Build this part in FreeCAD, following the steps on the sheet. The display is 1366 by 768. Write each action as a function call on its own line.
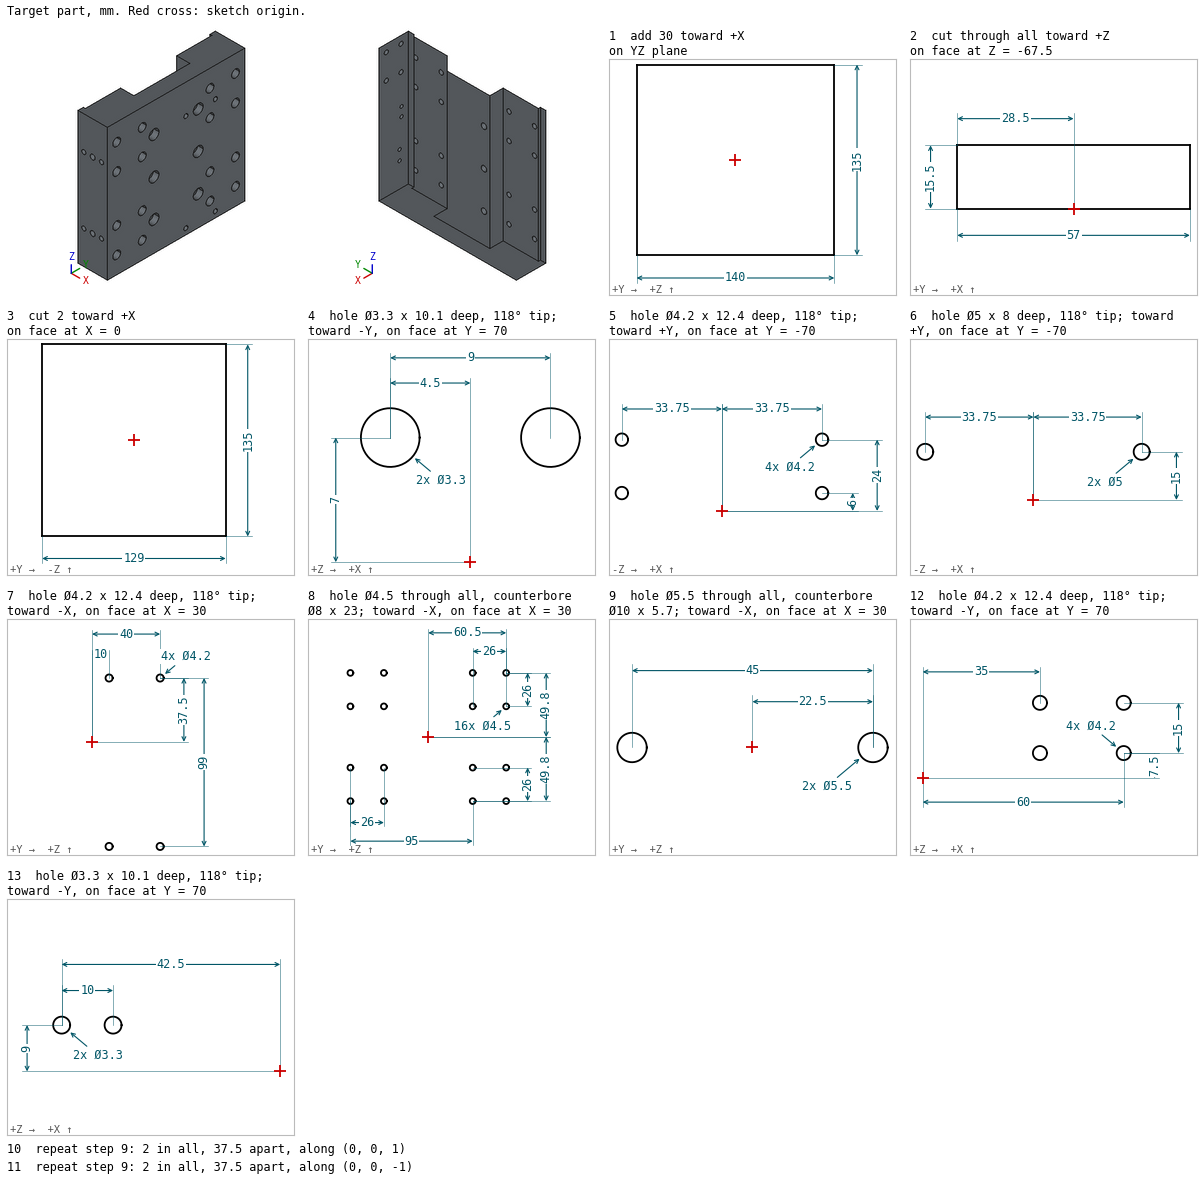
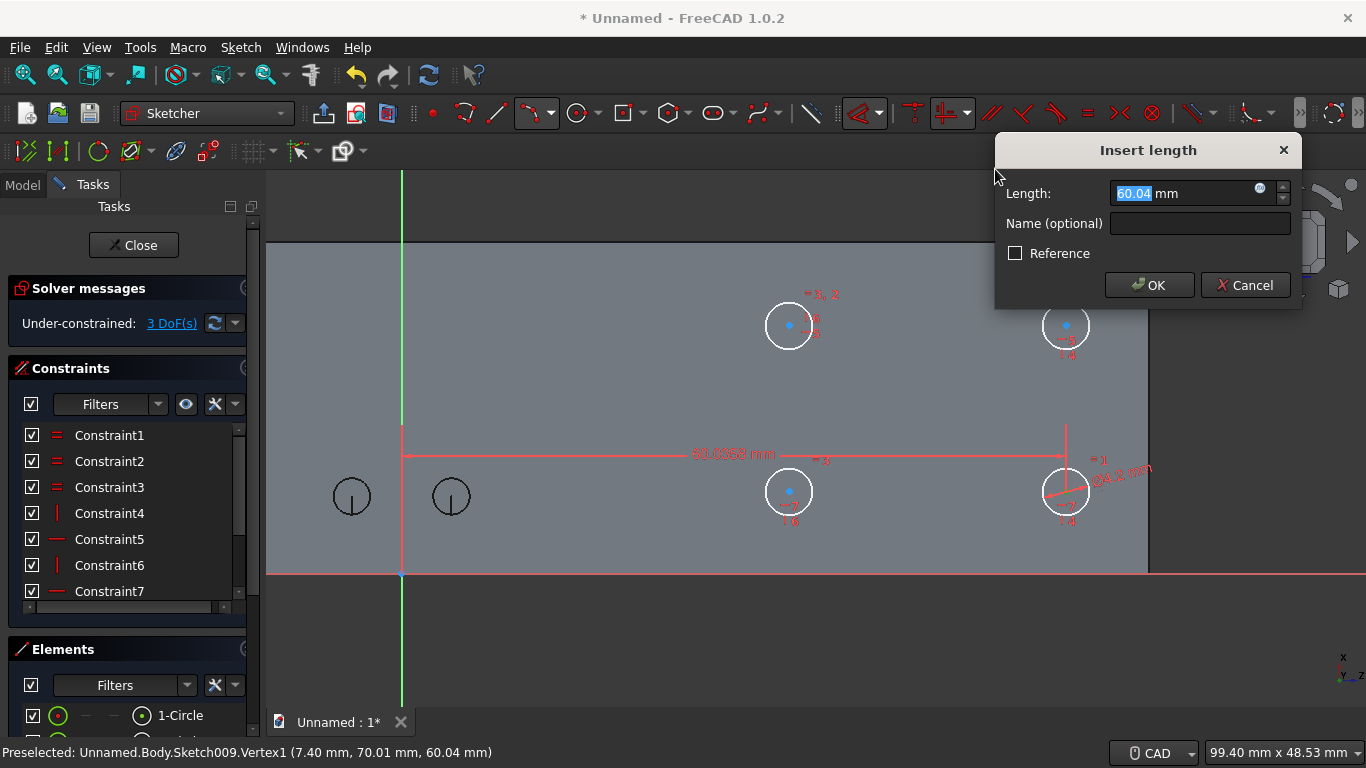
text(60)
key(Return)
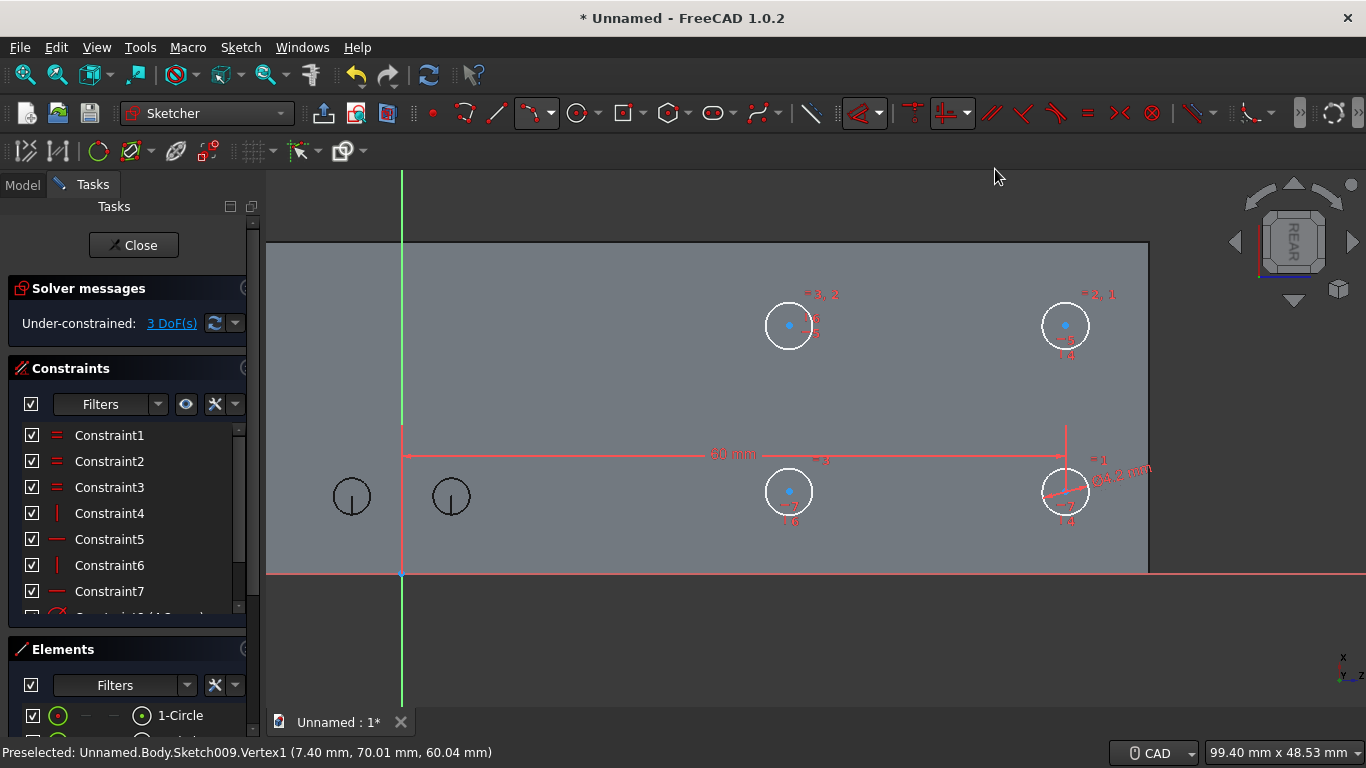
click(789, 326)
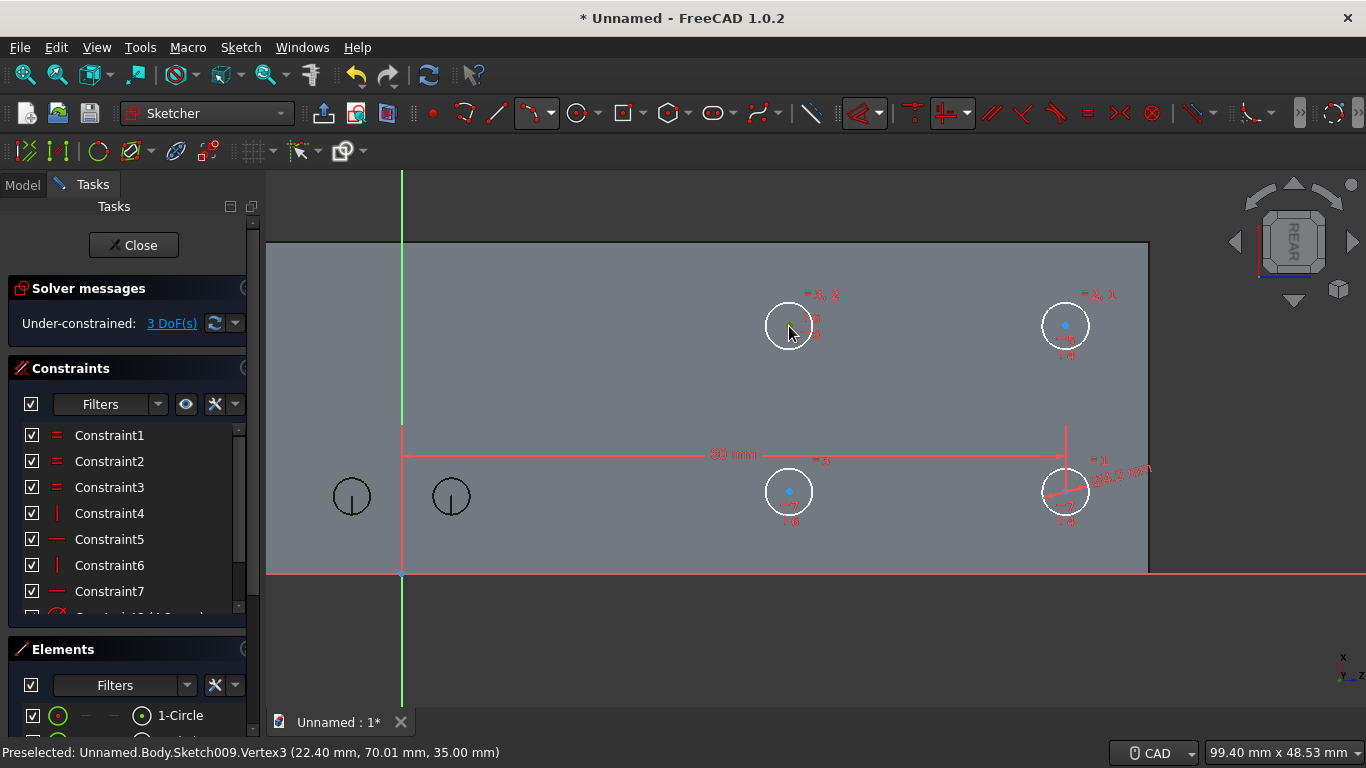
key(l)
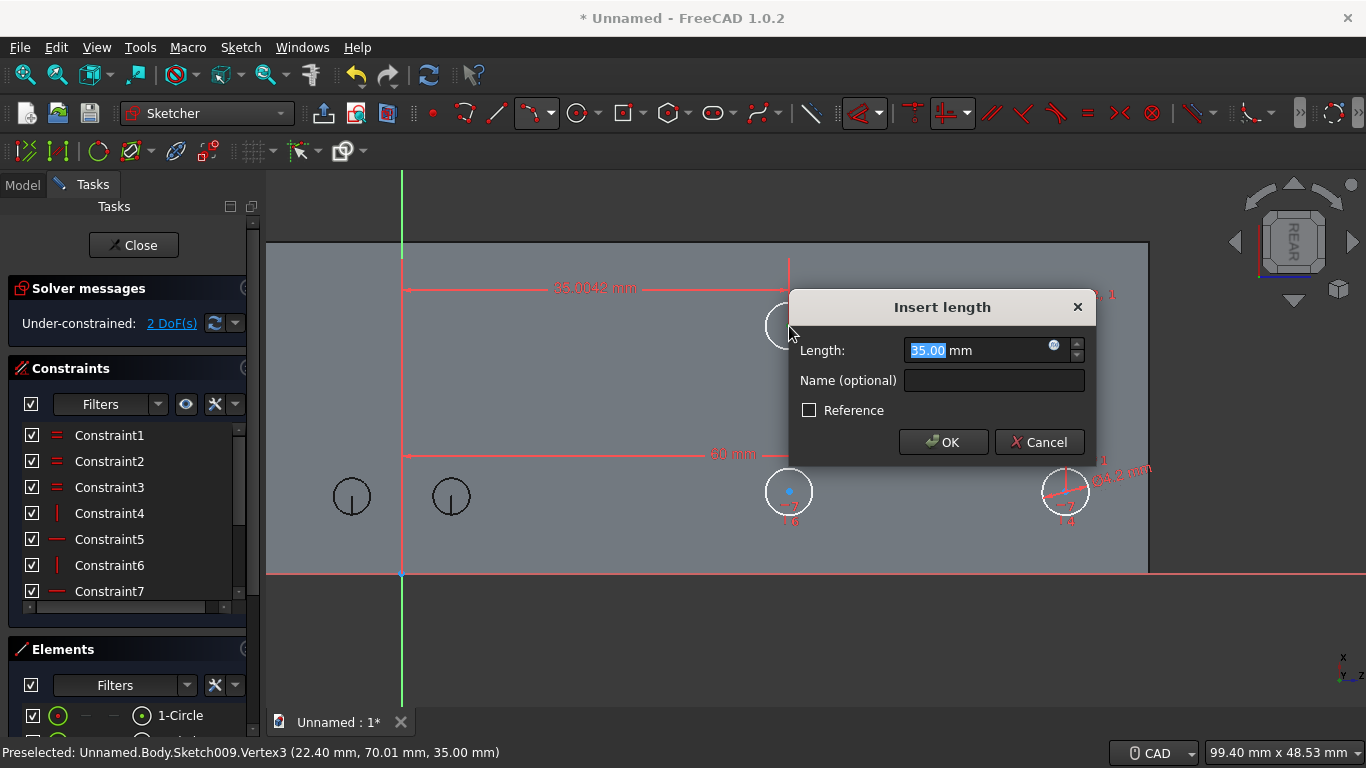
text(35)
key(Return)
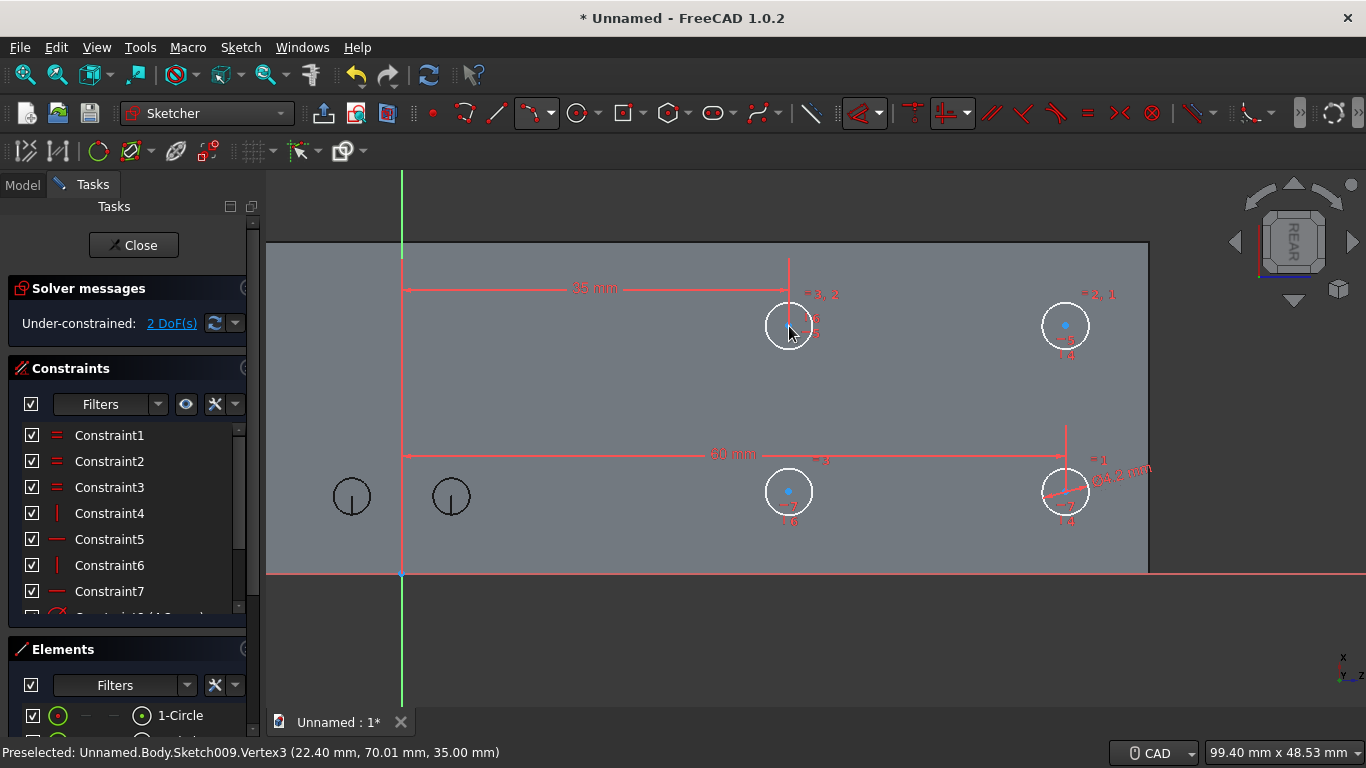
click(1066, 492)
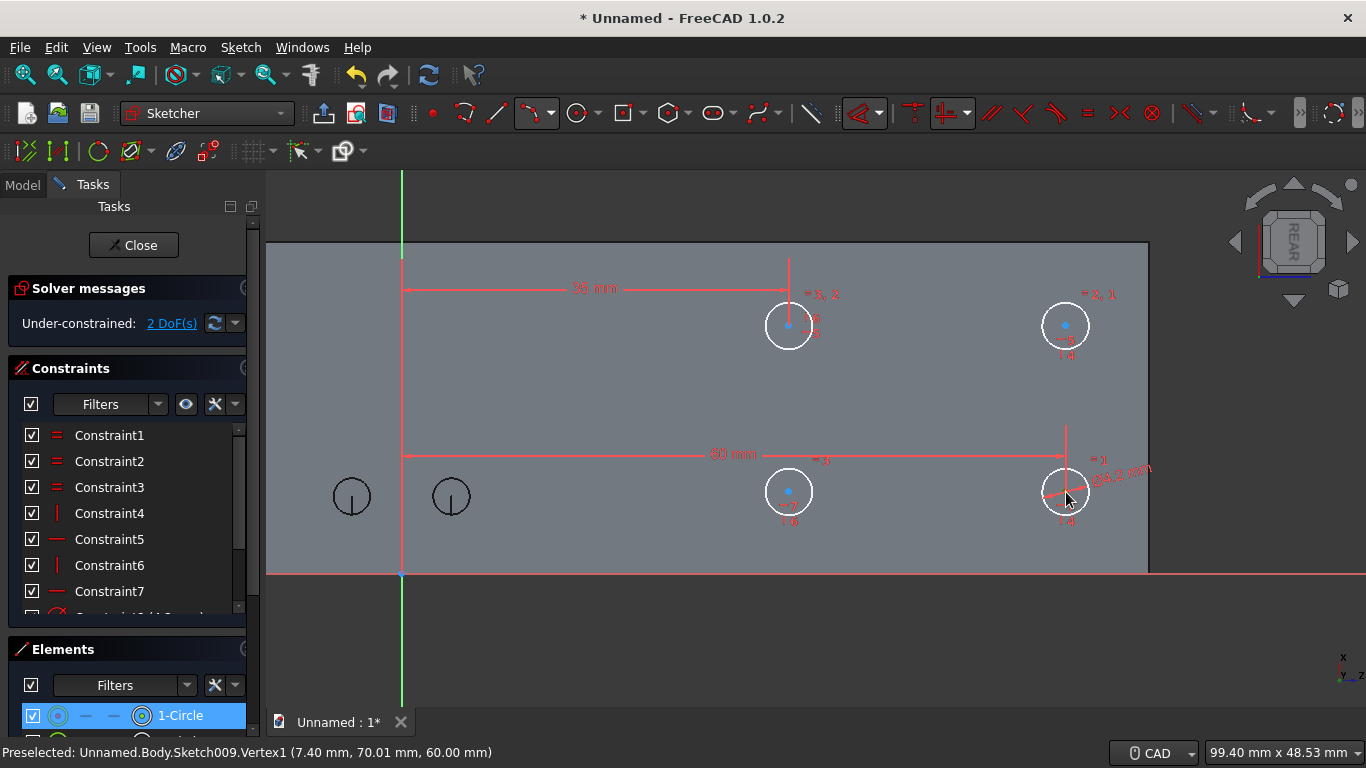
click(882, 114)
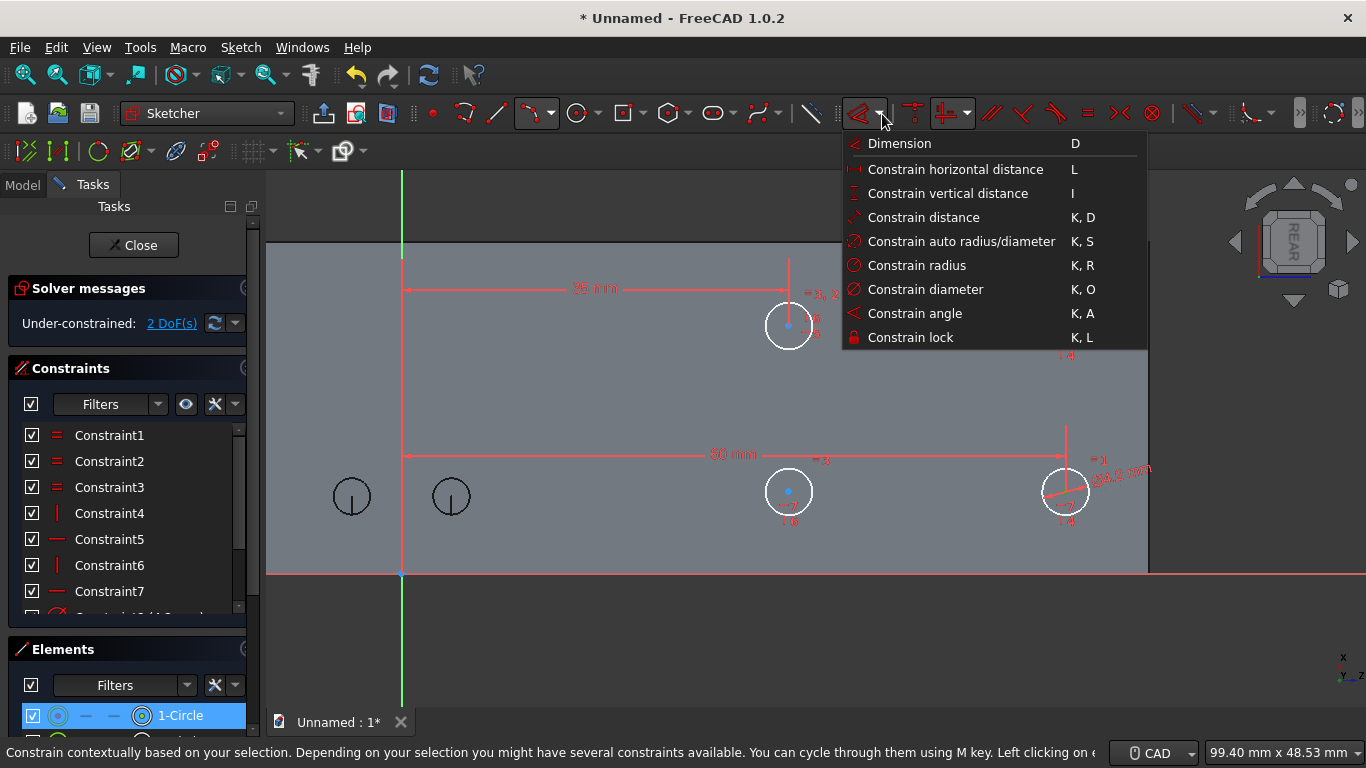
click(995, 193)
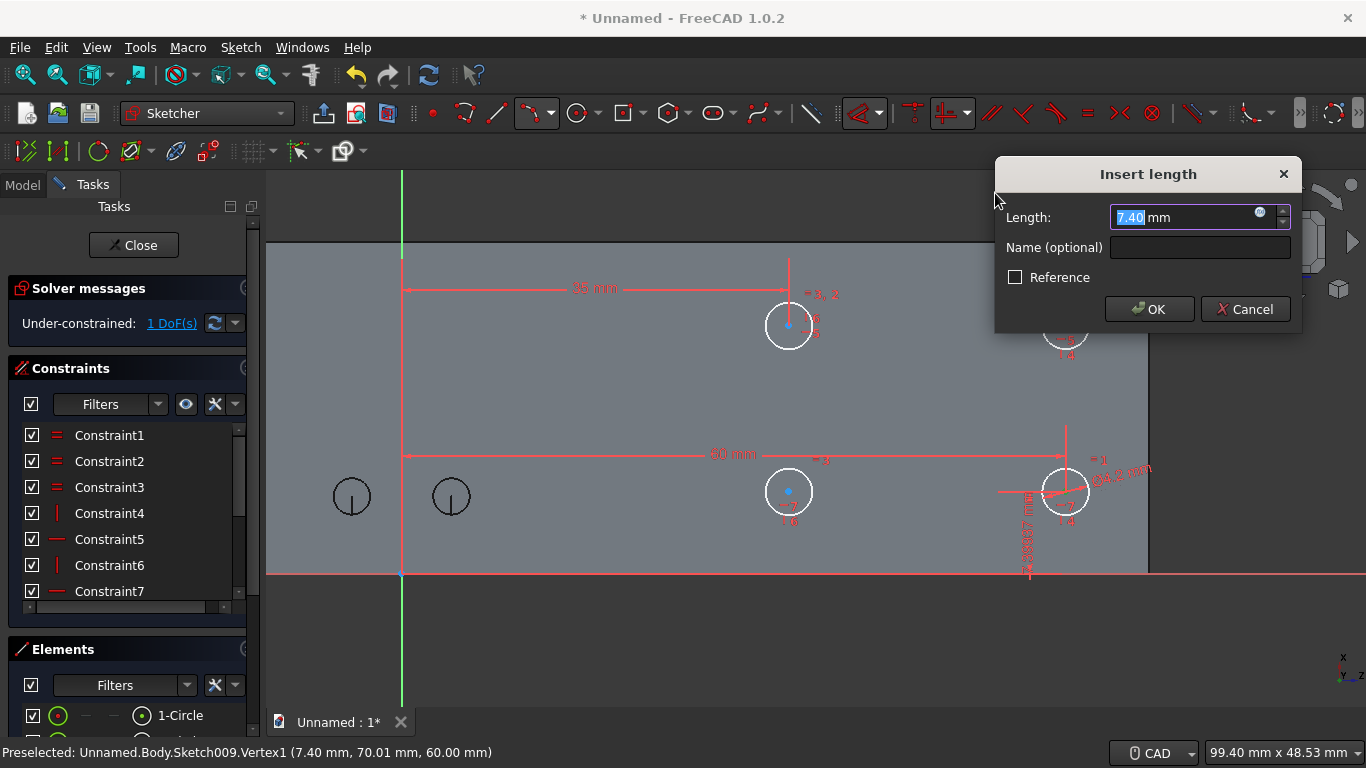
text(7.5)
key(Return)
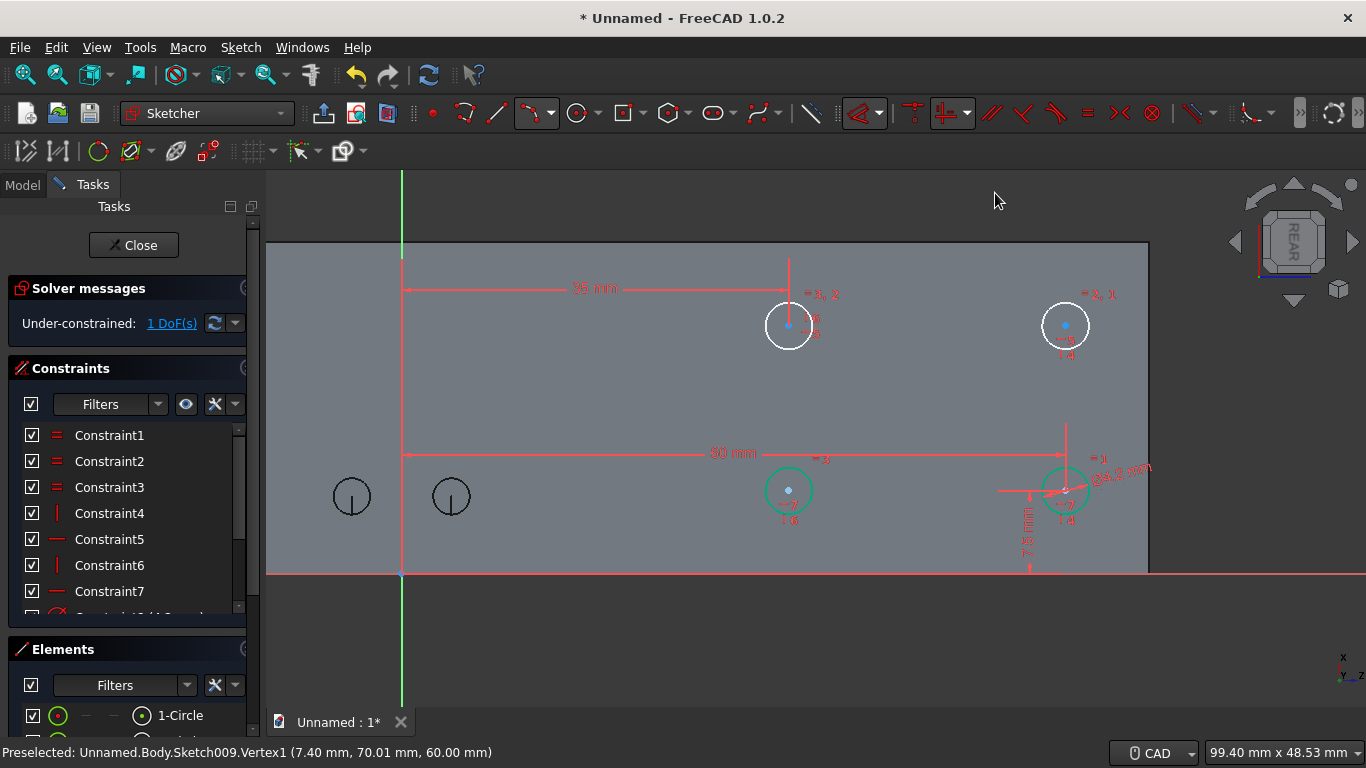
click(1066, 491)